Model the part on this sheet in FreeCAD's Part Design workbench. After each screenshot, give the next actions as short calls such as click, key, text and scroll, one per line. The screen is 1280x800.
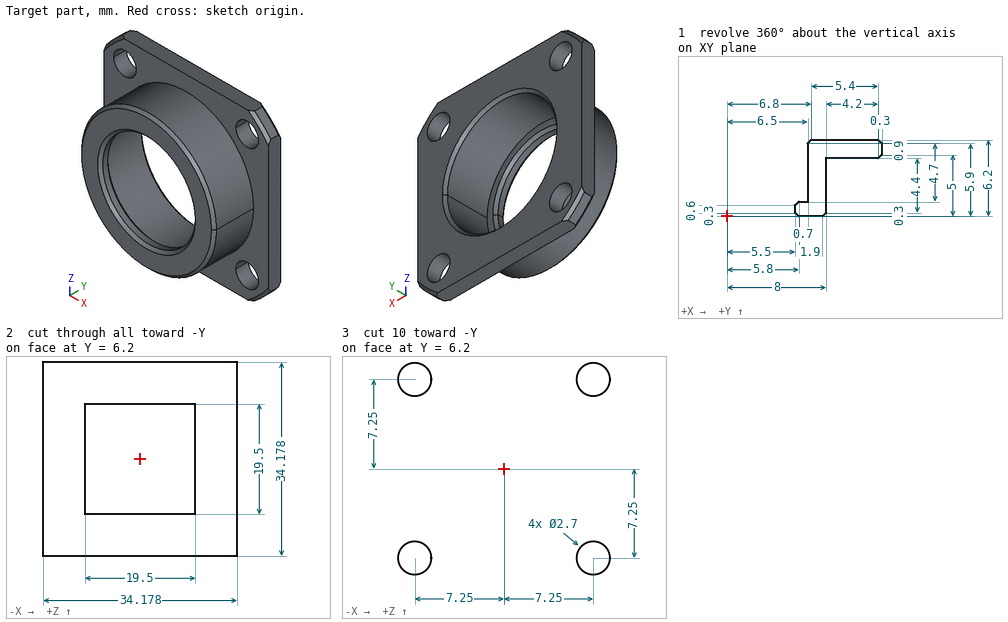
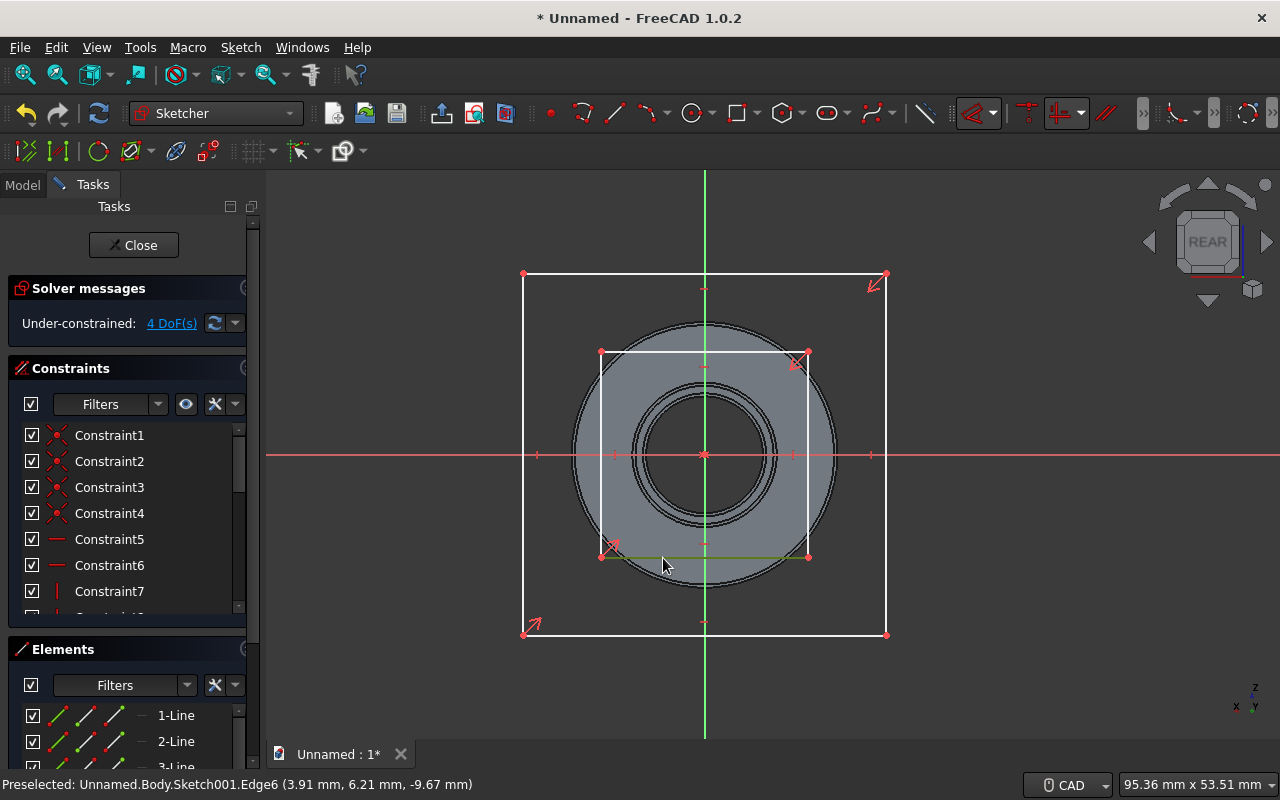
click(996, 114)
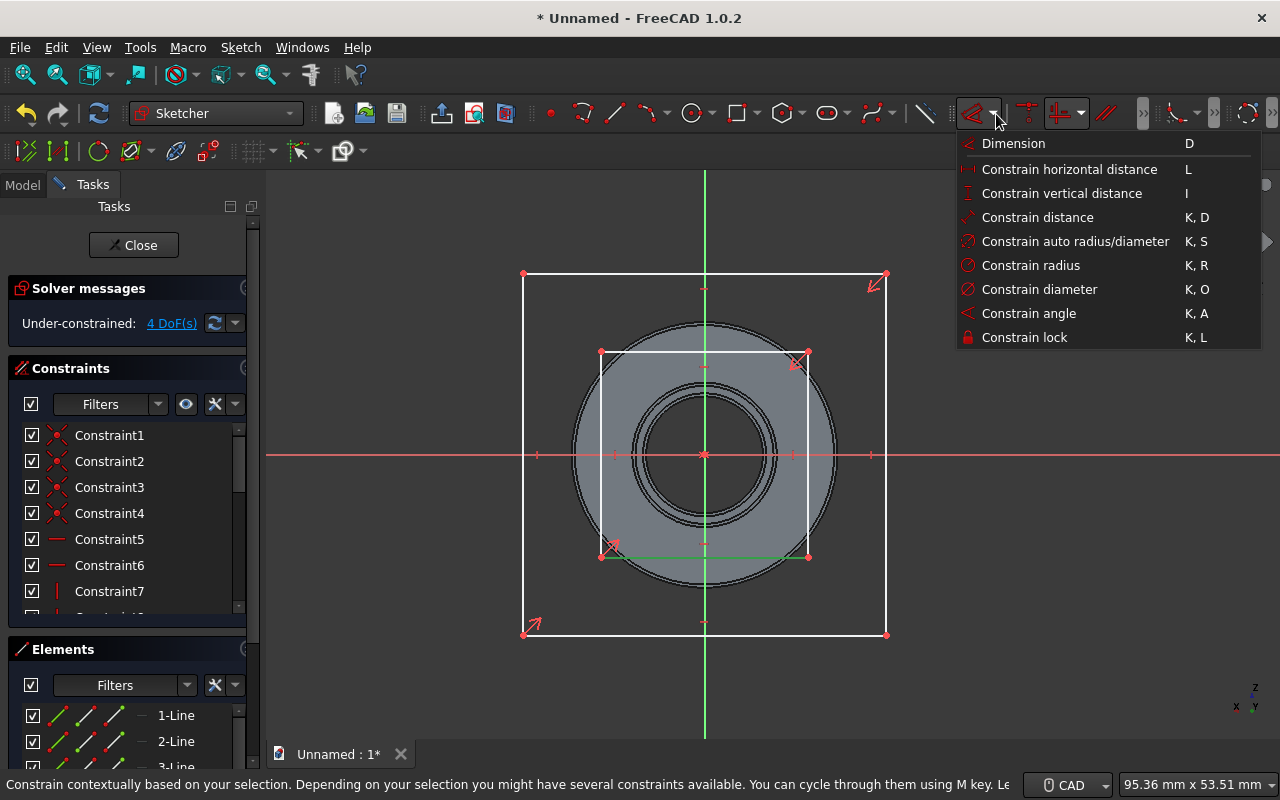
click(1109, 169)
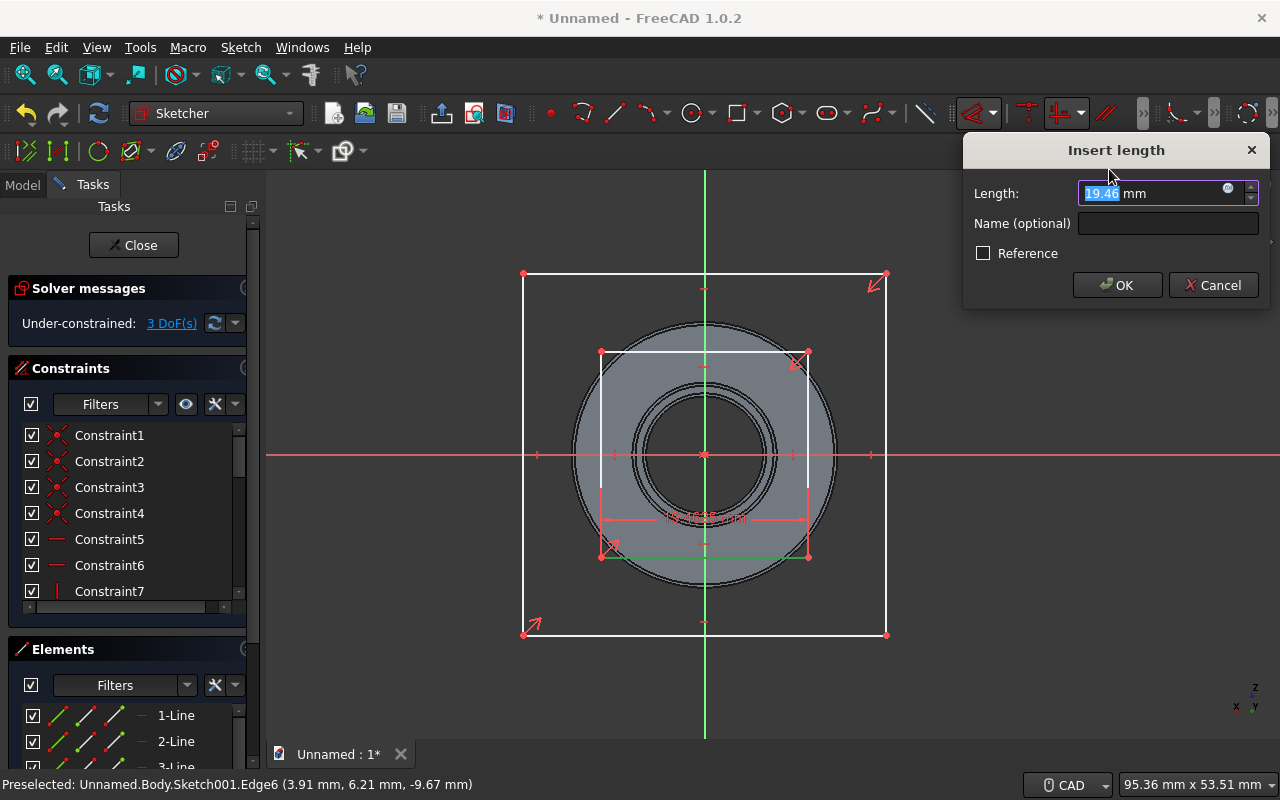
text(19.5)
key(Return)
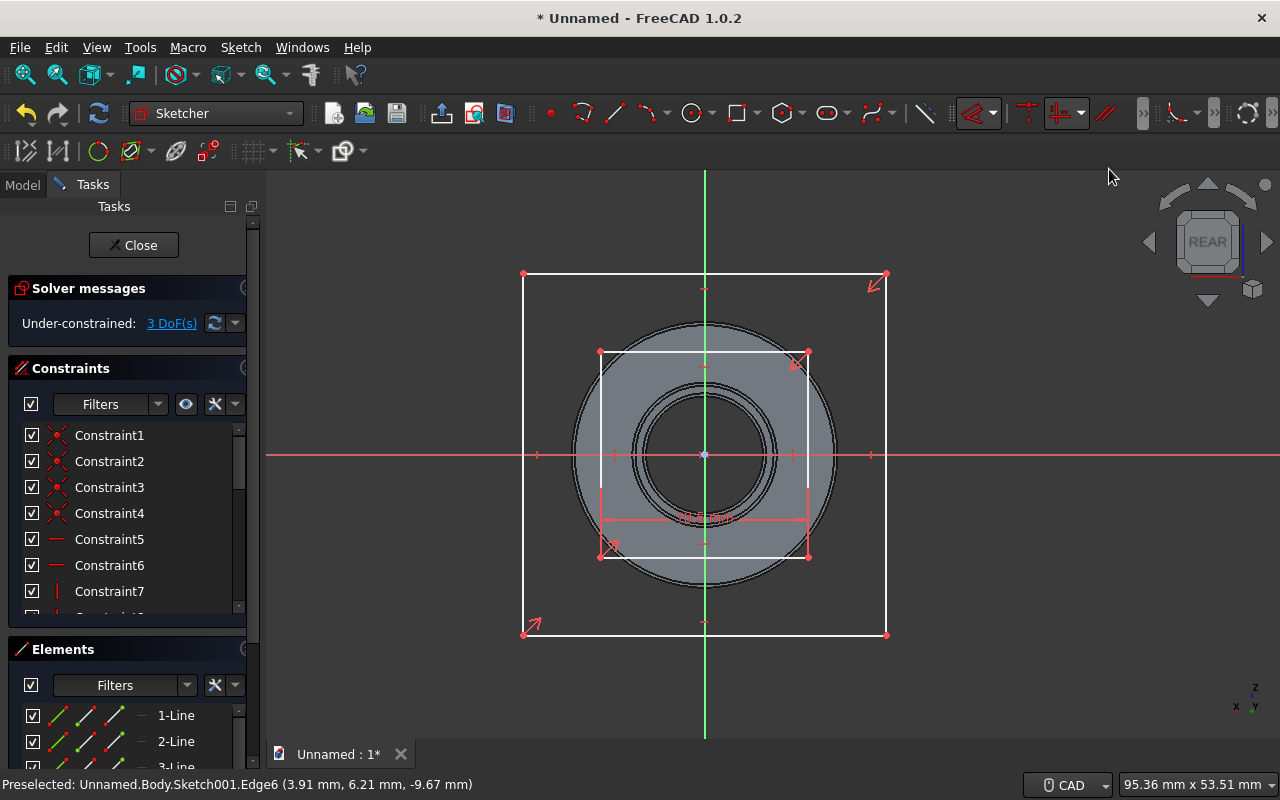
click(808, 496)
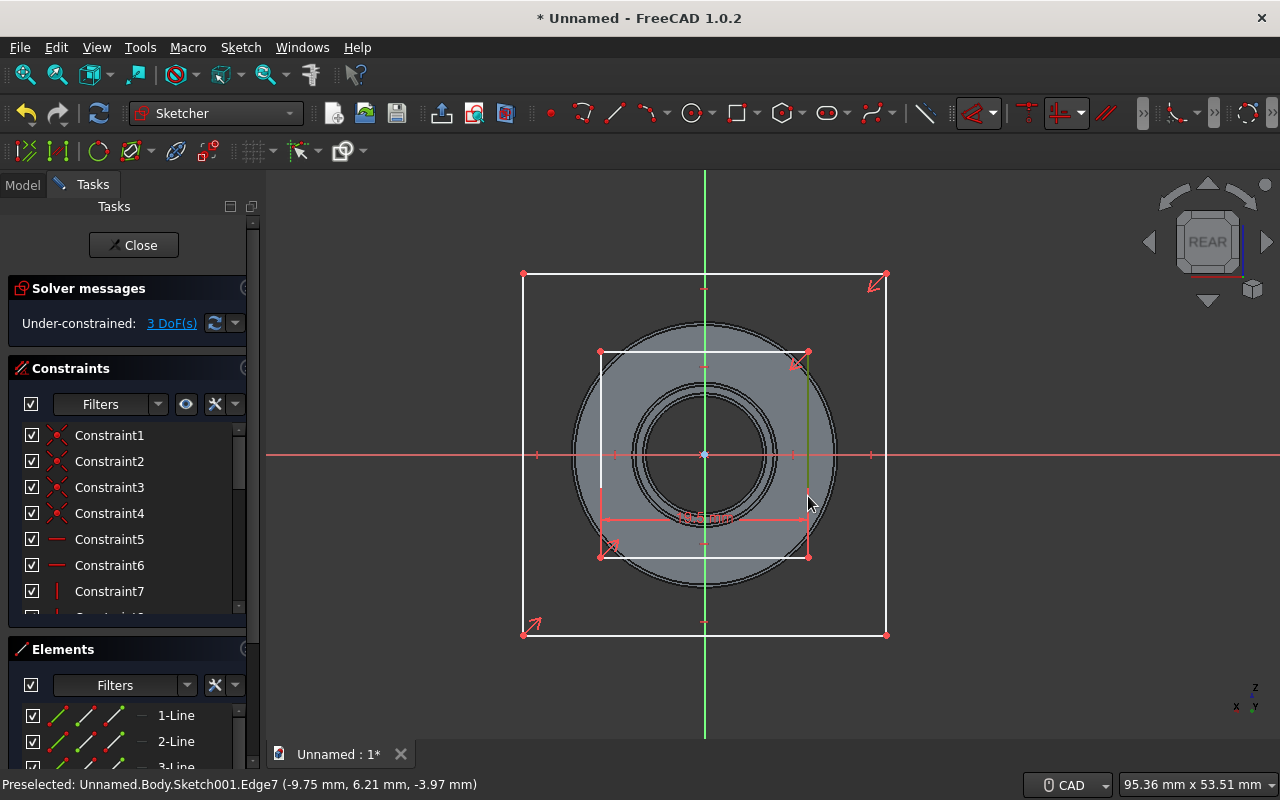
click(996, 114)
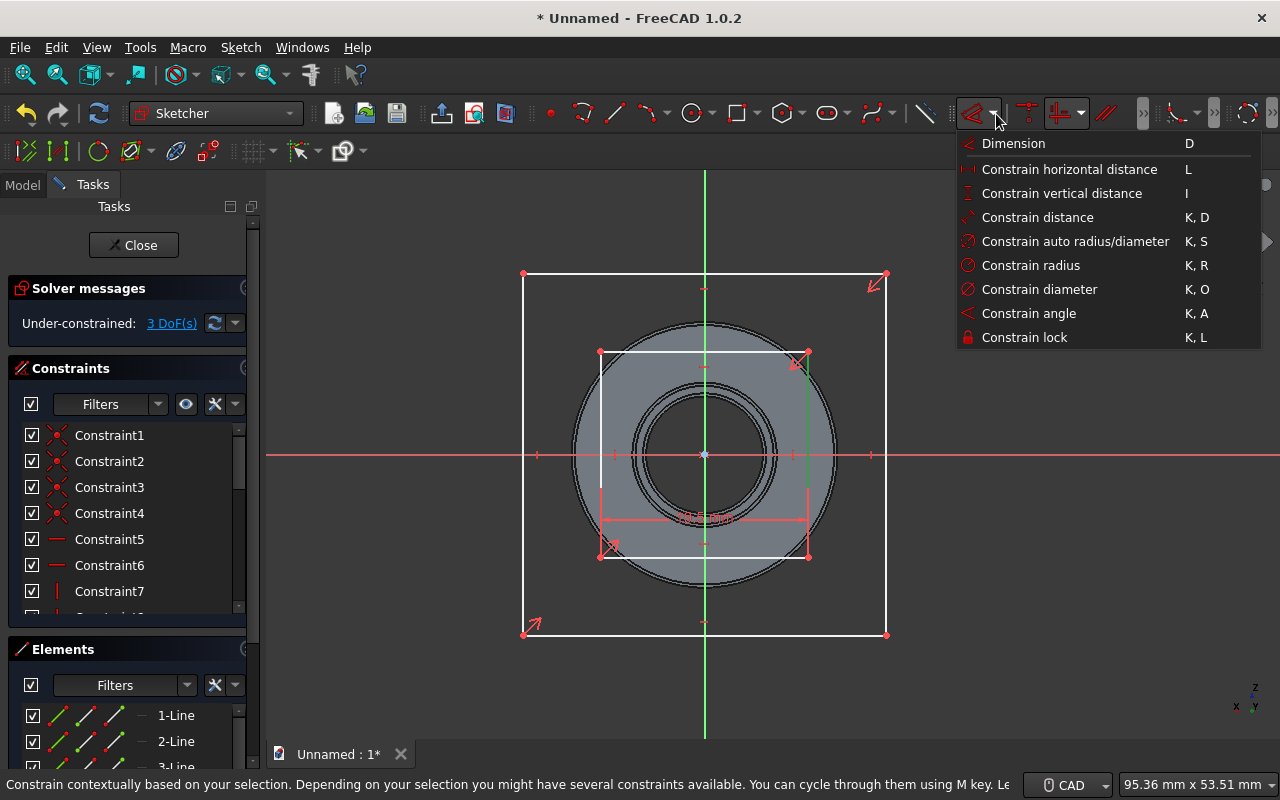
click(1109, 193)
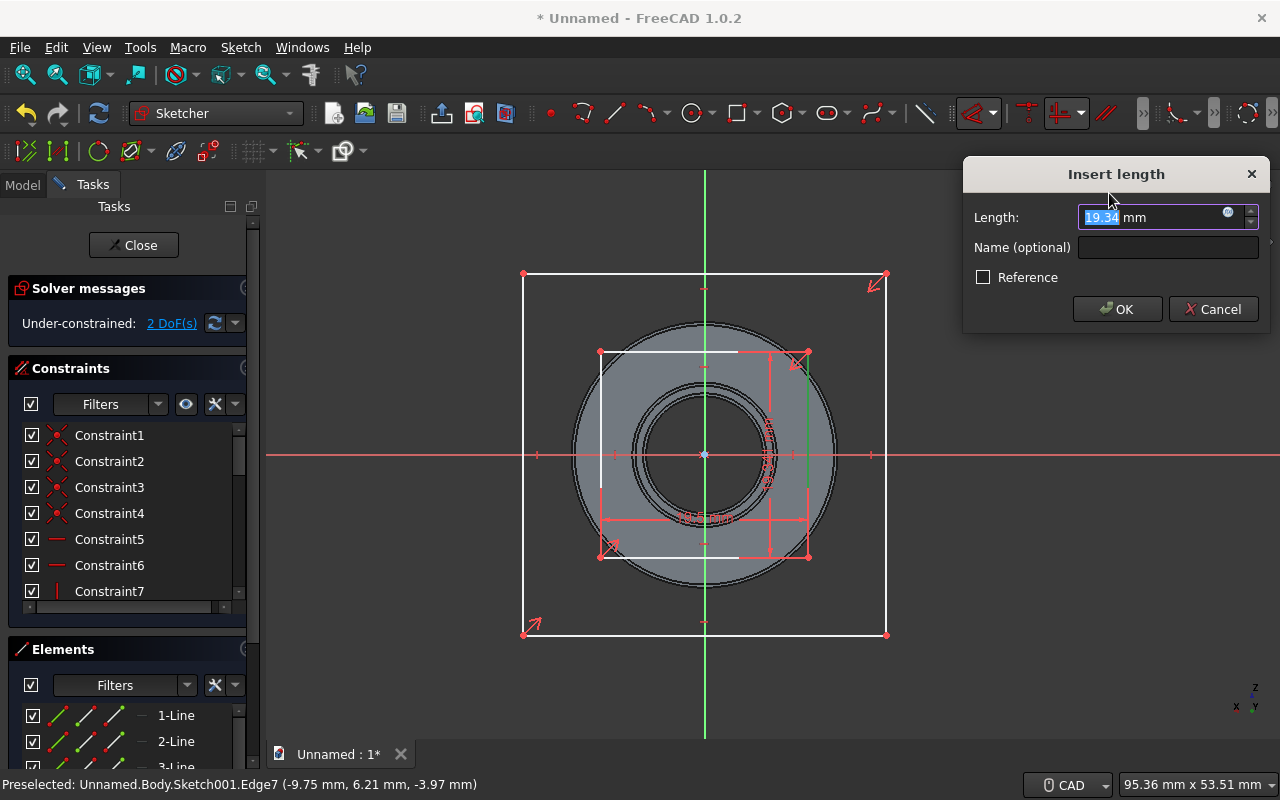
text(19.5)
key(Return)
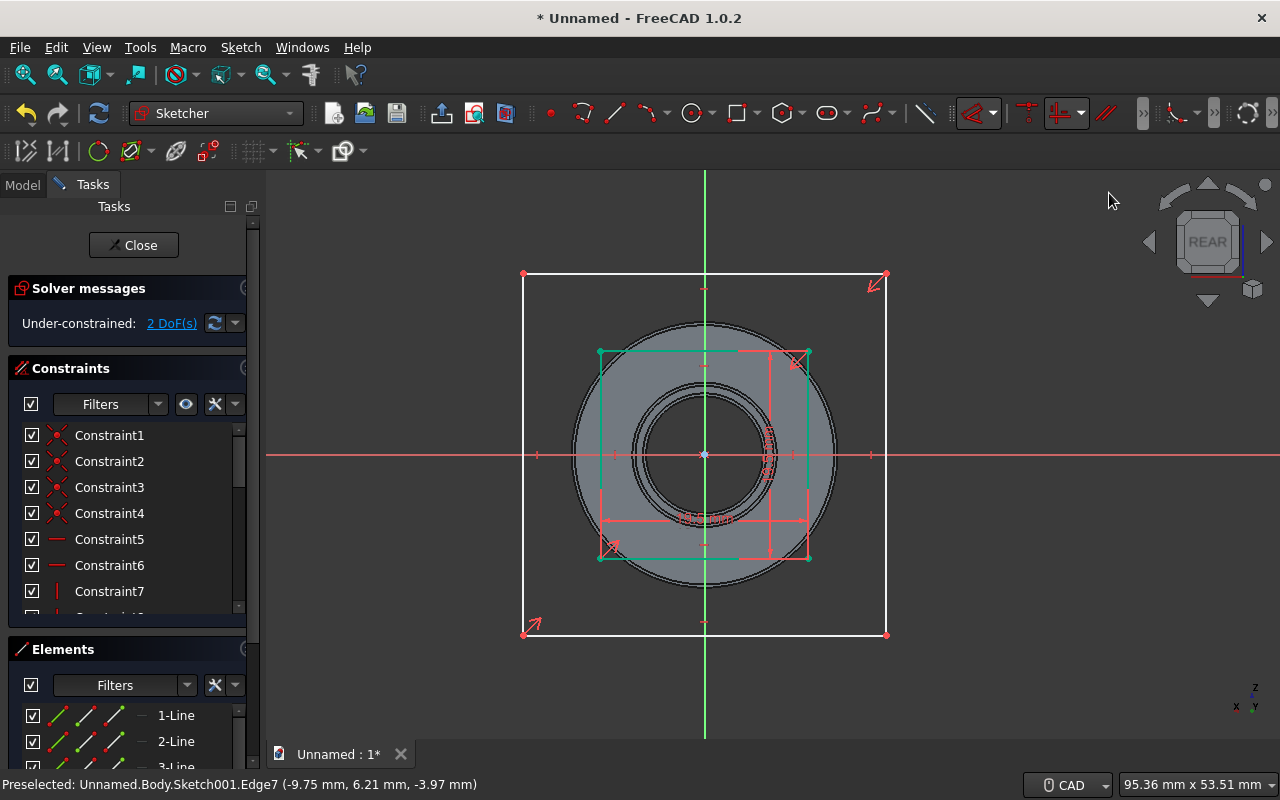
click(632, 636)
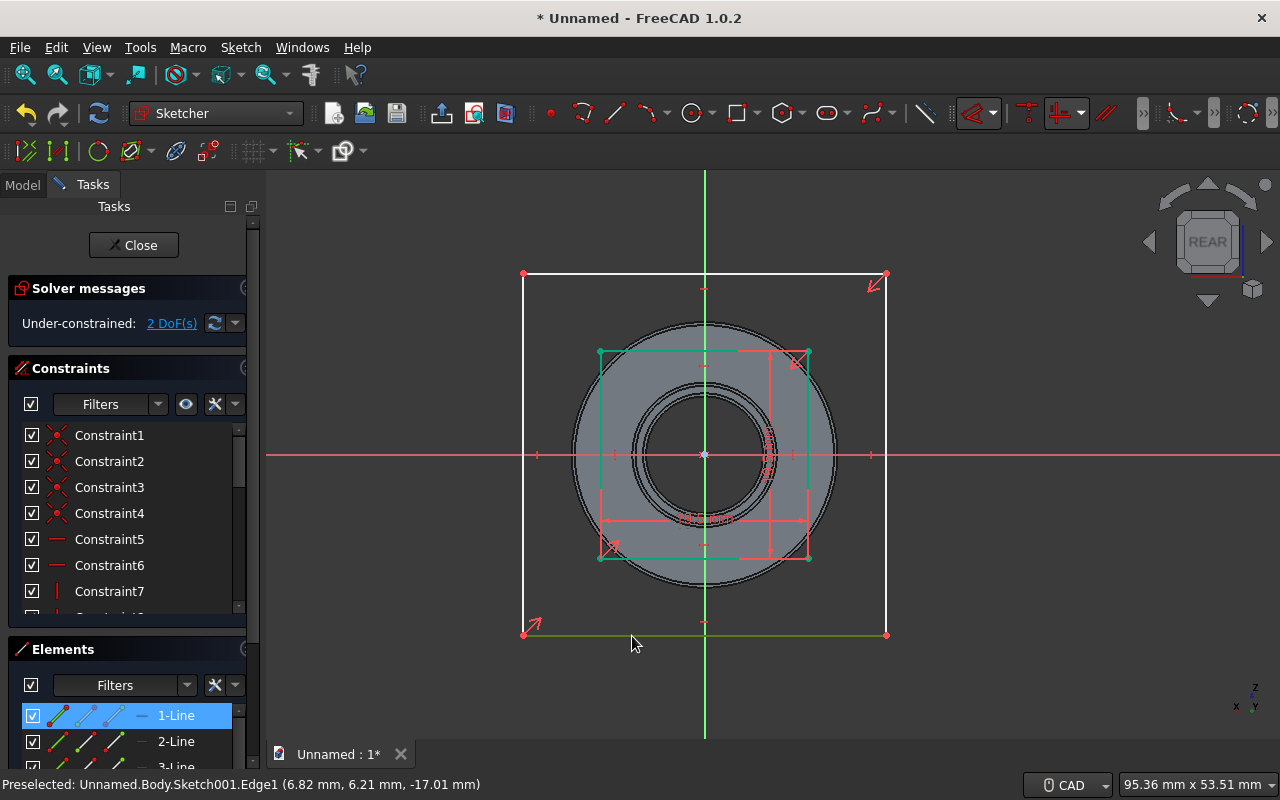
key(l)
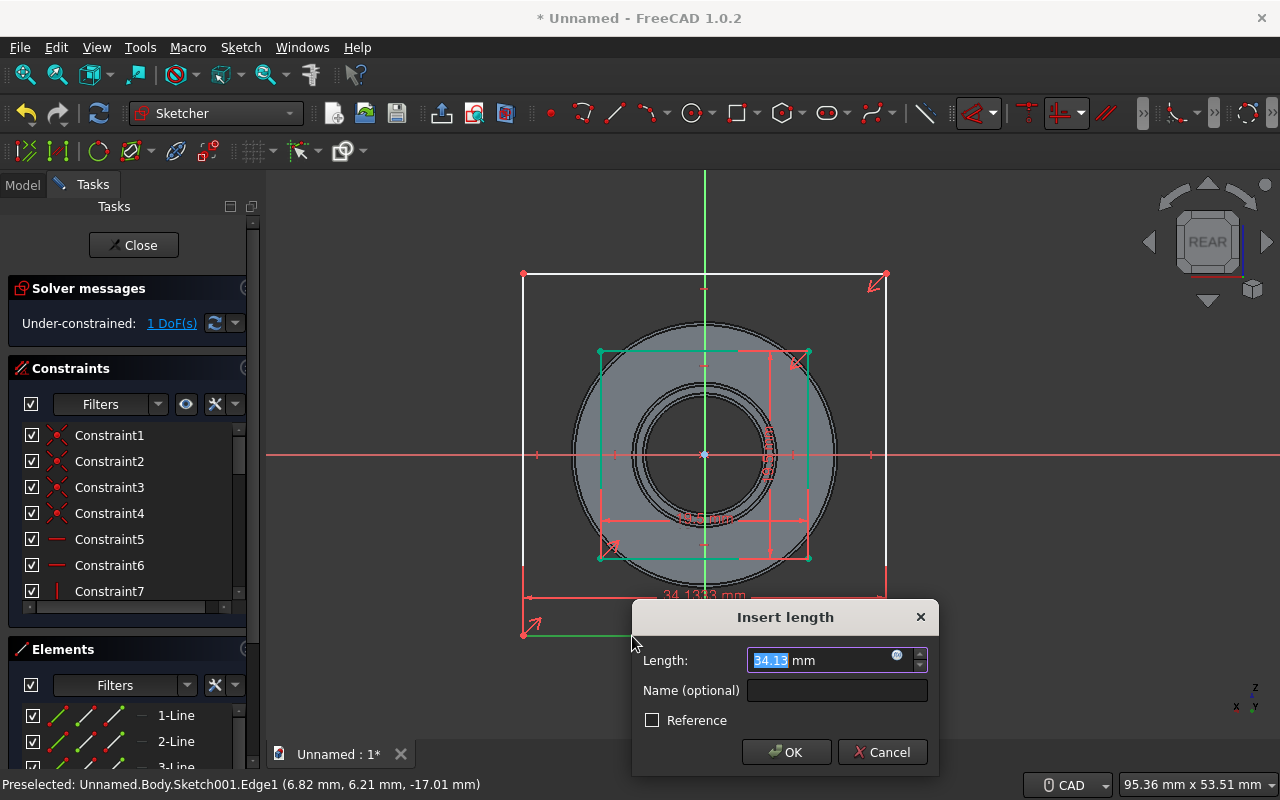
text(34.178)
key(Return)